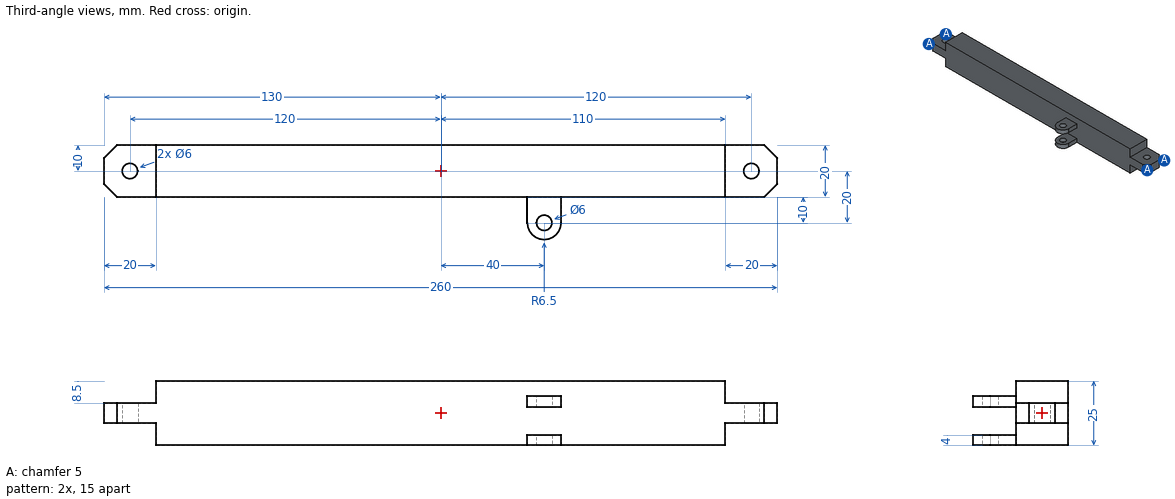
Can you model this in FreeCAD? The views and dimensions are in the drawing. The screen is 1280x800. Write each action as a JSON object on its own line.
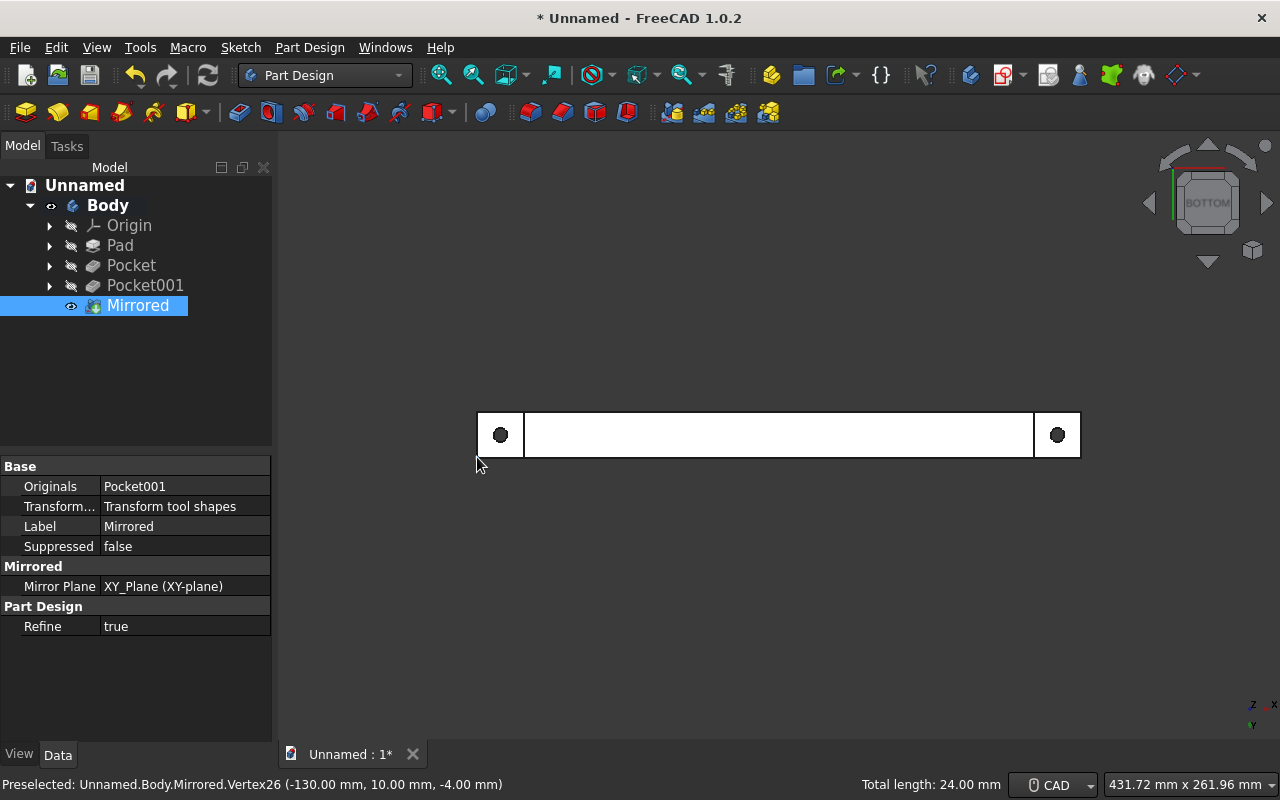
{"action": "key", "text": "4"}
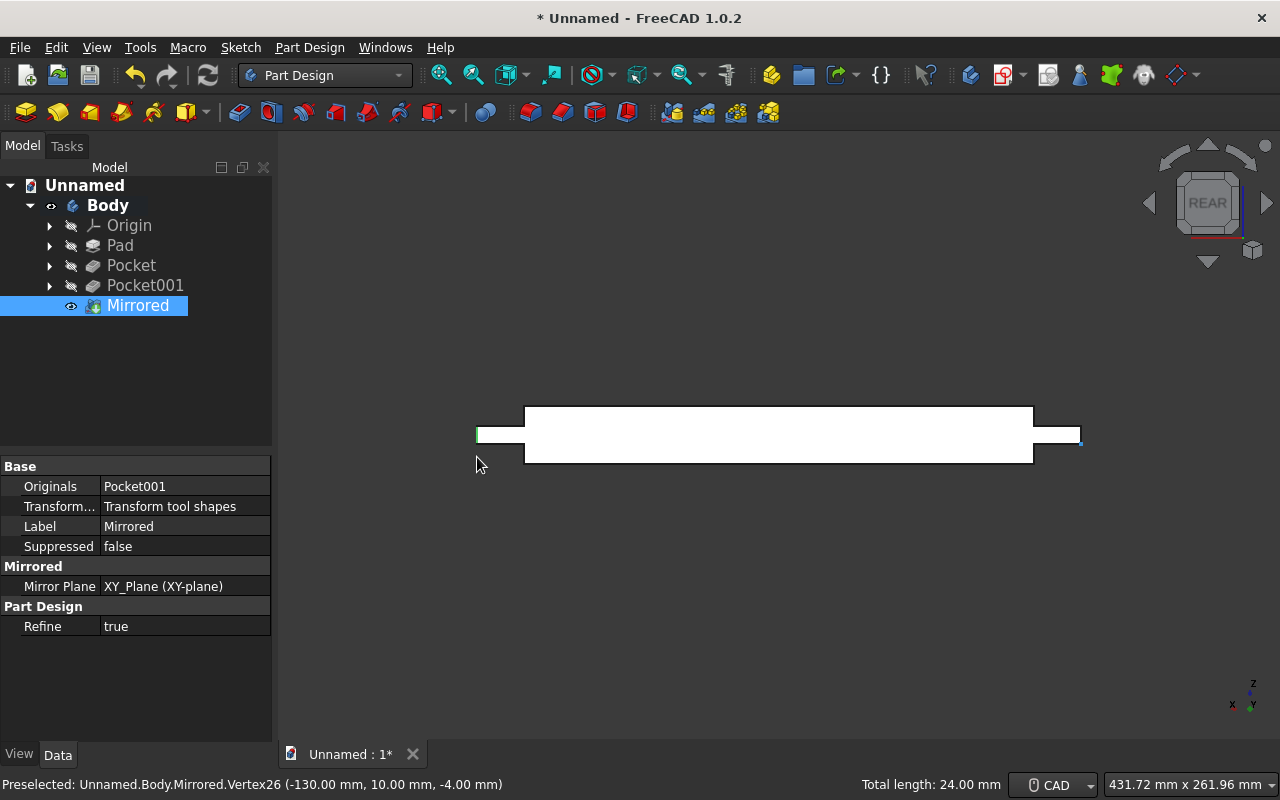
{"action": "left_click", "coordinate": [1081, 434], "text": "ctrl"}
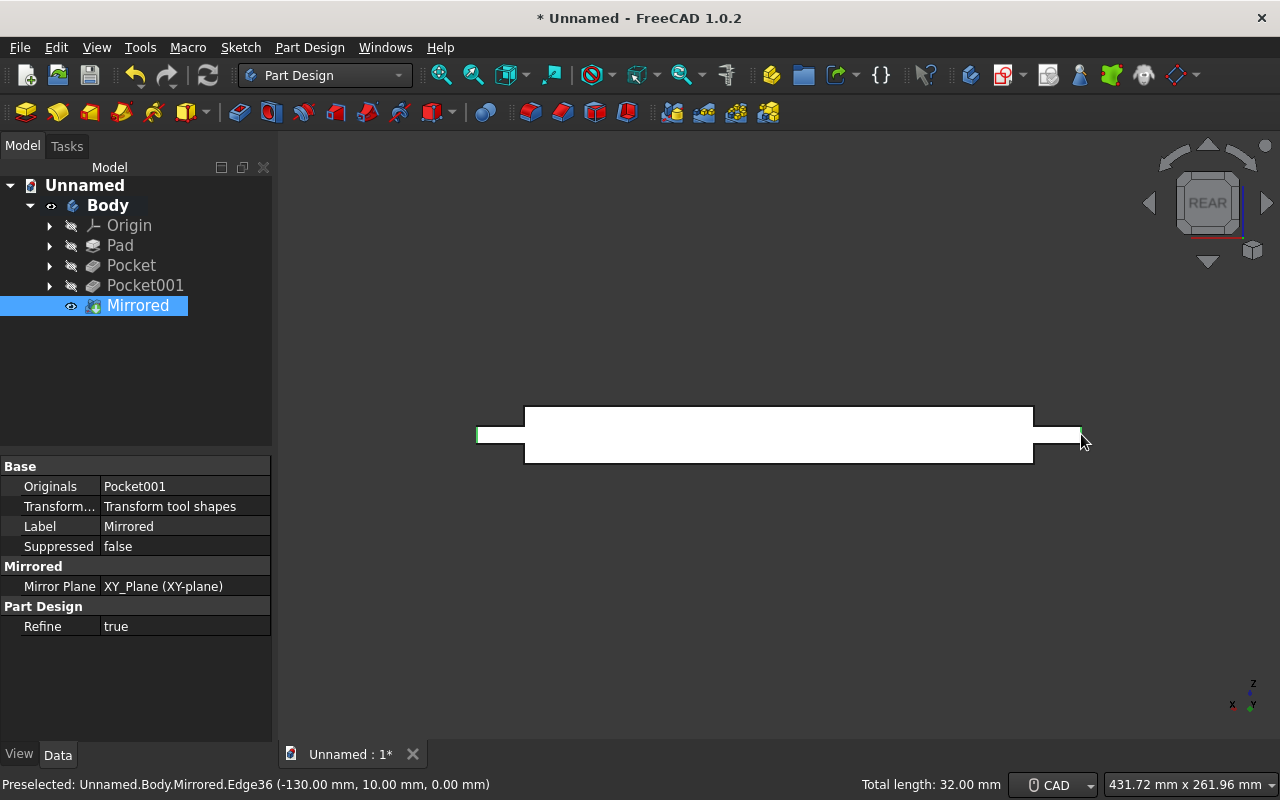
{"action": "left_click", "coordinate": [564, 112]}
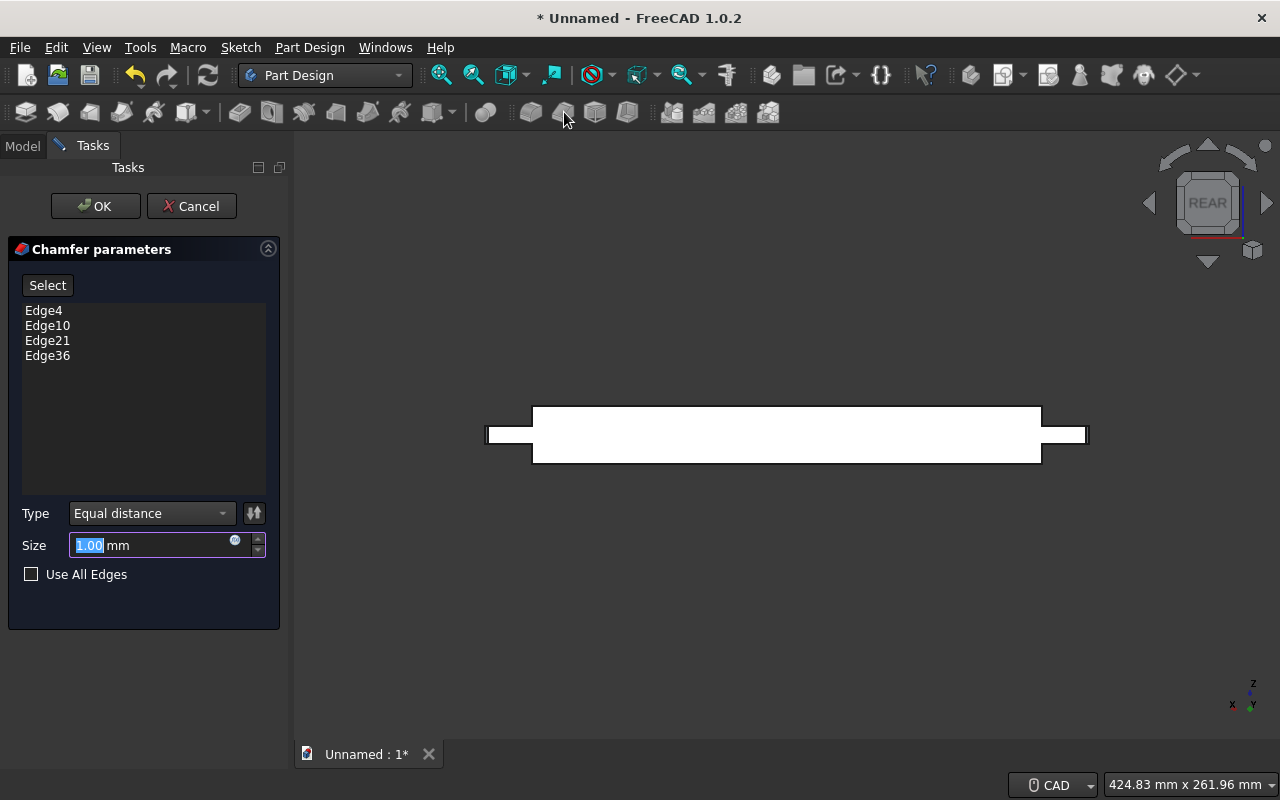
{"action": "type", "text": "5"}
{"action": "key", "text": "Tab"}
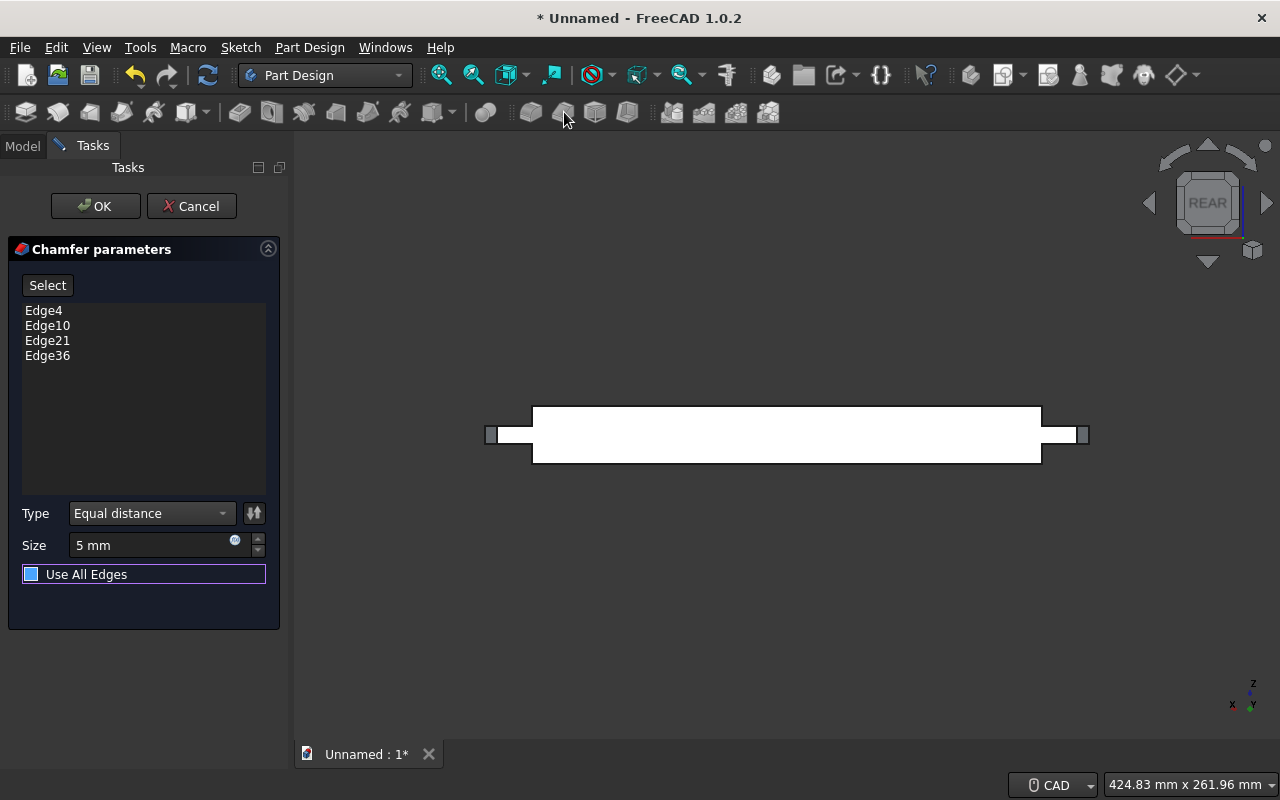
{"action": "left_click", "coordinate": [96, 206]}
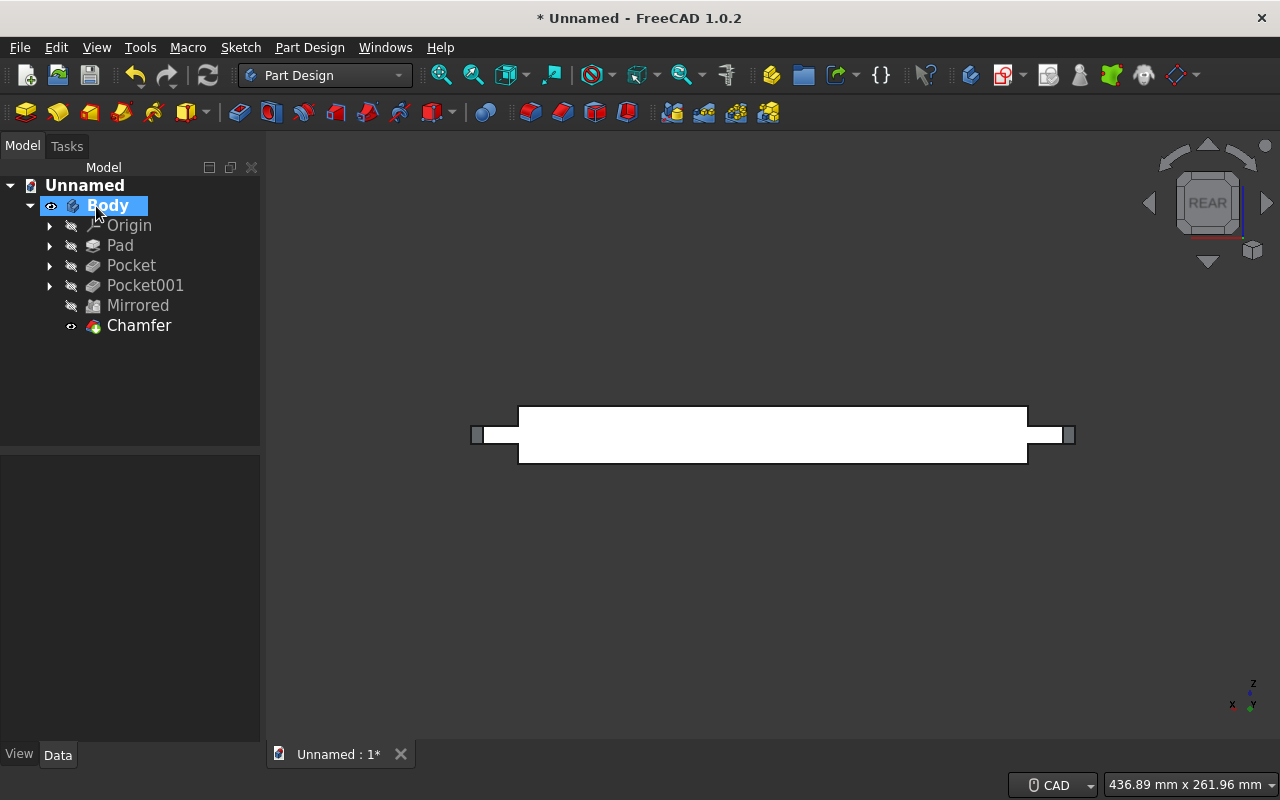
{"action": "key", "text": "5"}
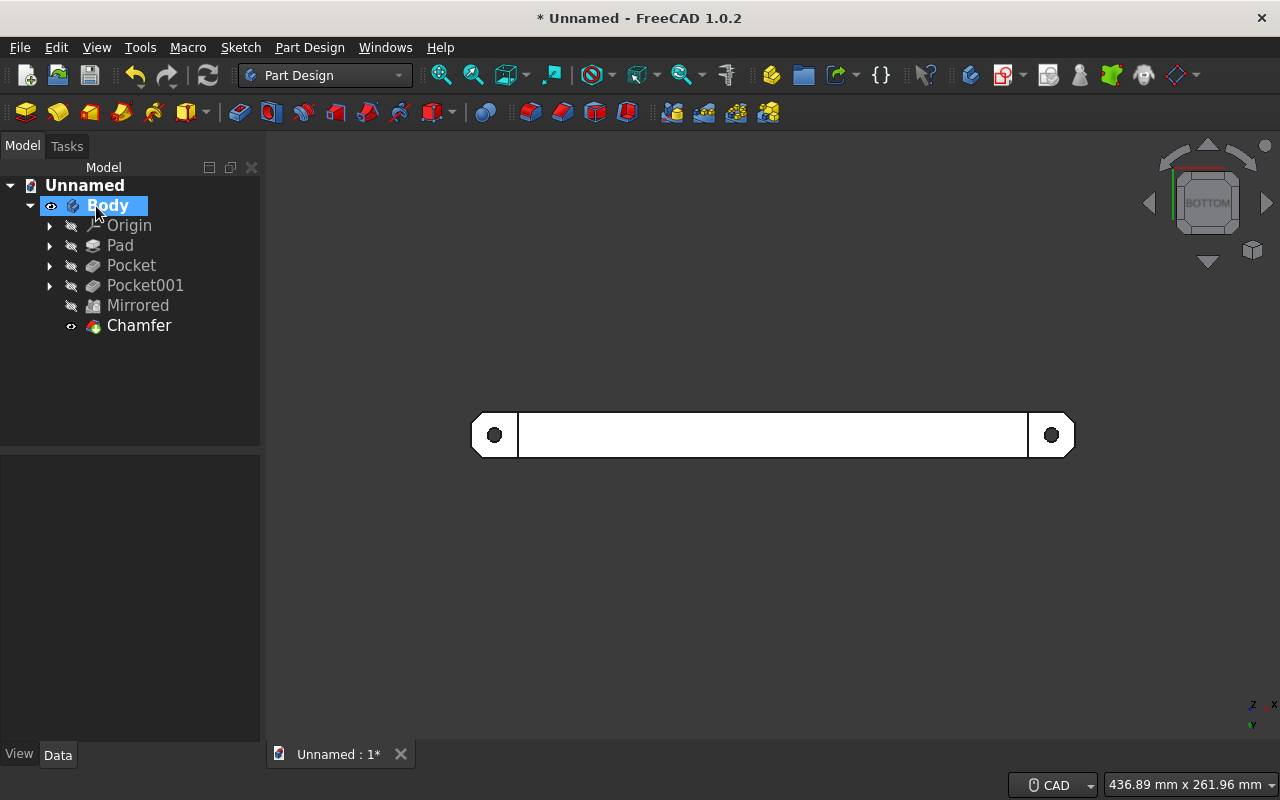
{"action": "left_click", "coordinate": [992, 434]}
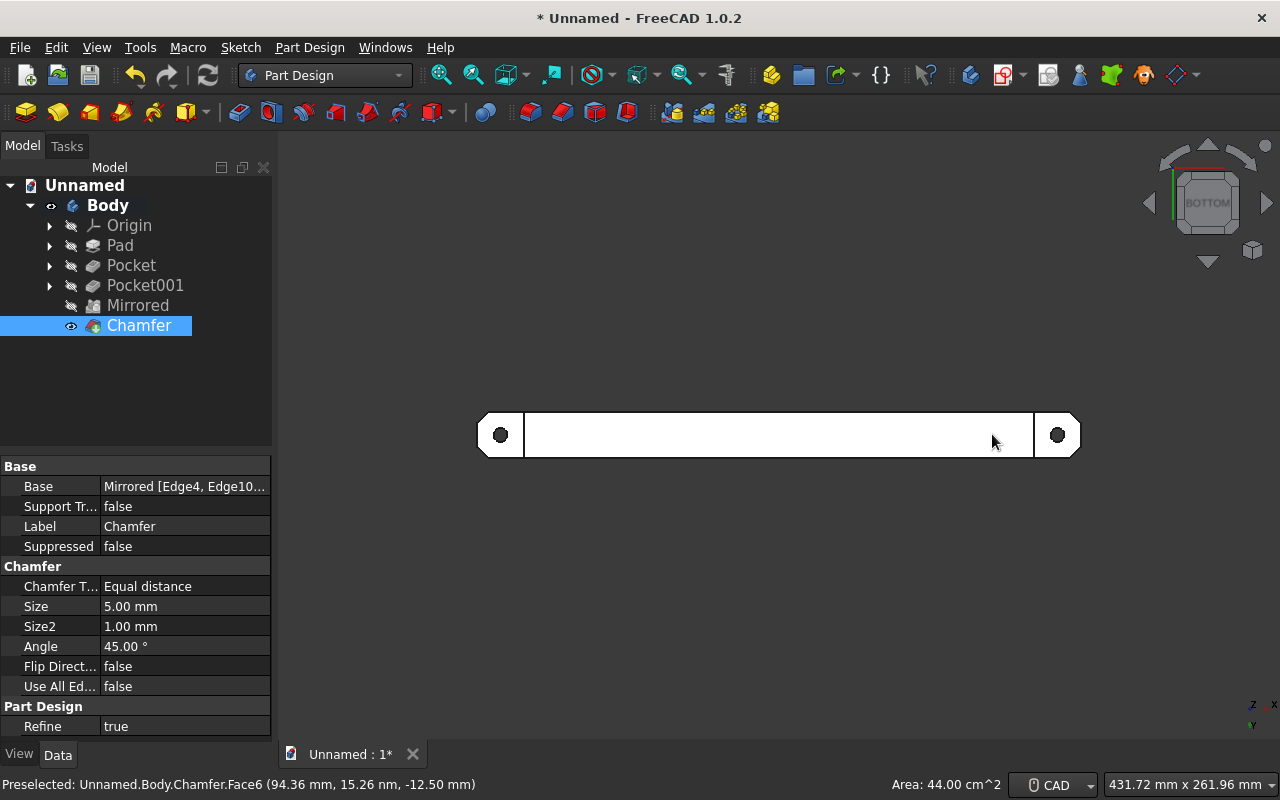
{"action": "left_click", "coordinate": [1004, 76]}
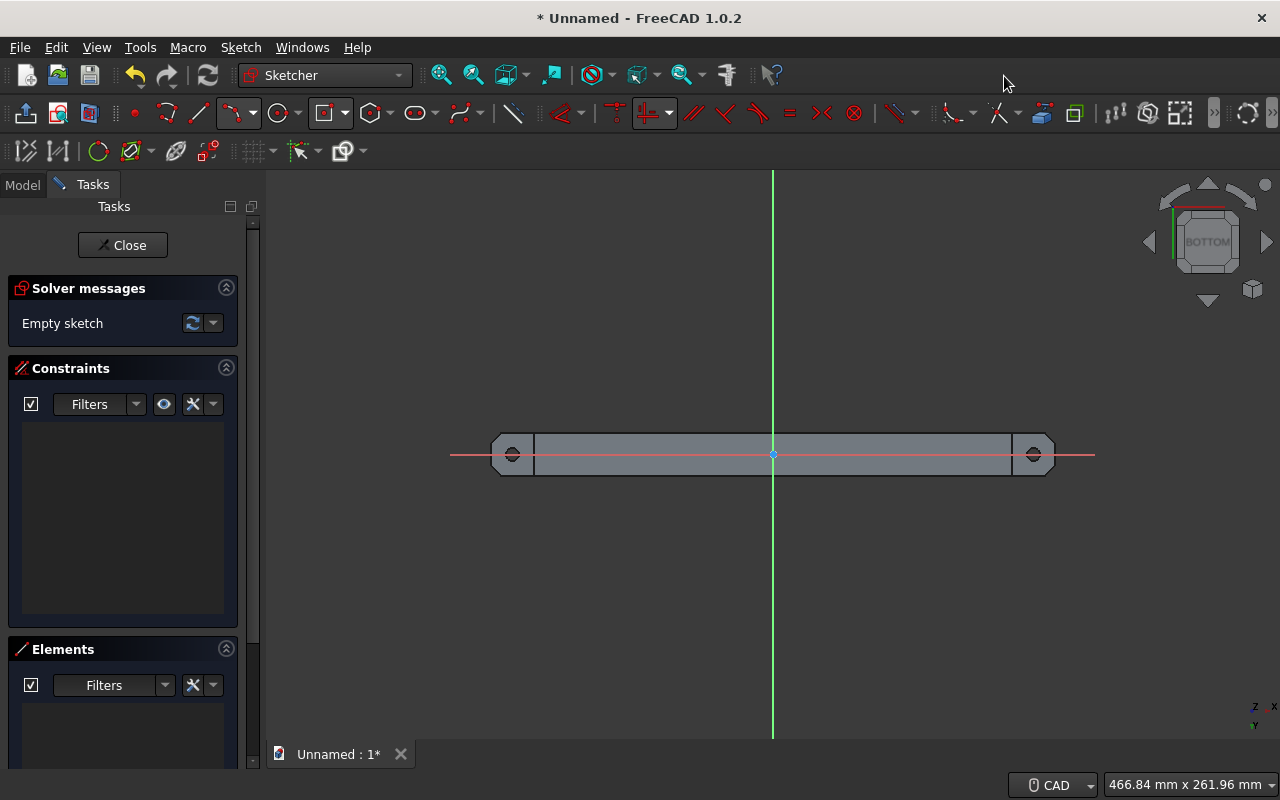
{"action": "scroll", "coordinate": [875, 411], "scroll_direction": "up", "scroll_amount": 12}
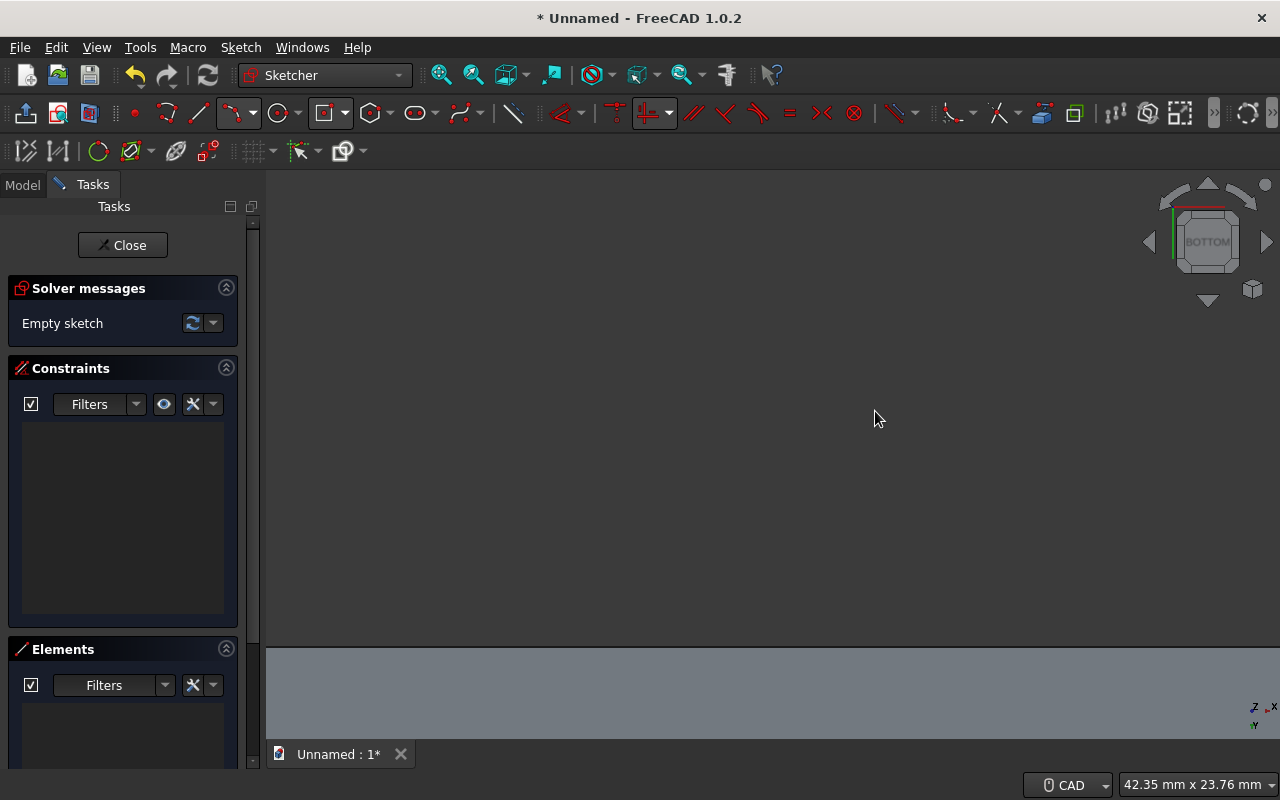
{"action": "key", "text": "g m"}